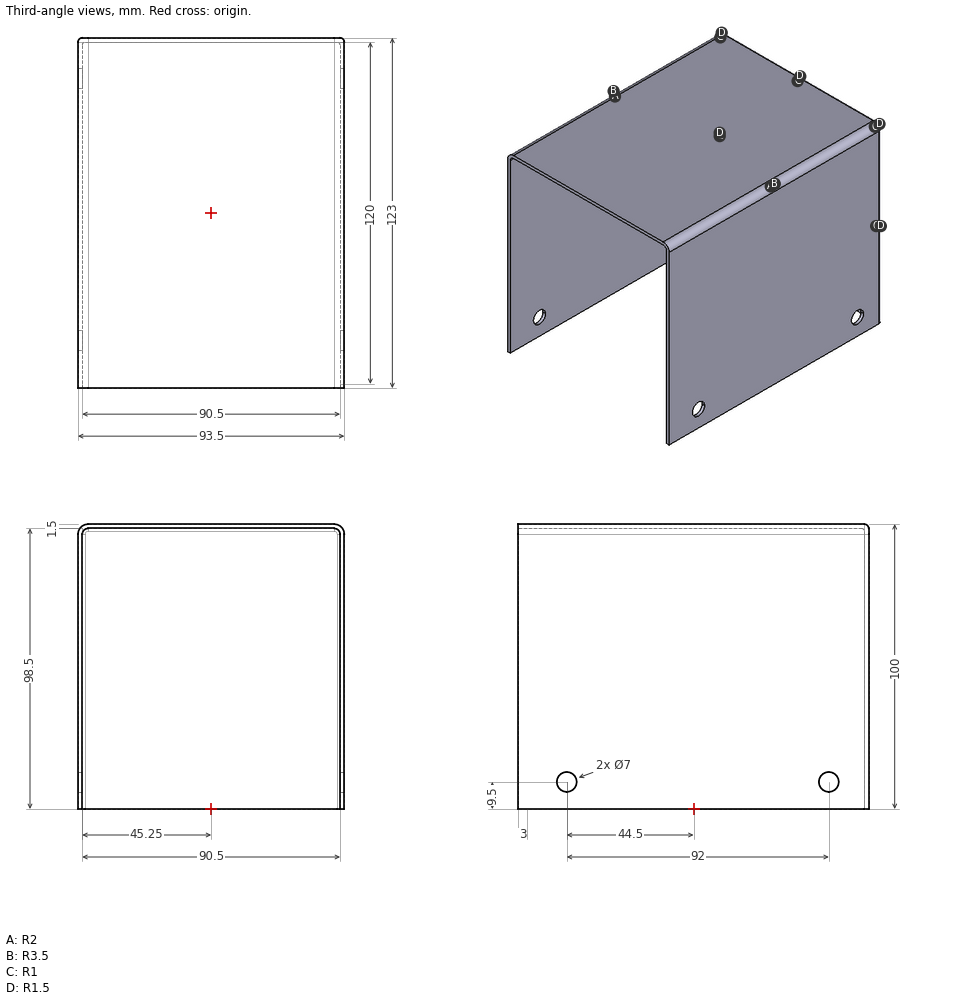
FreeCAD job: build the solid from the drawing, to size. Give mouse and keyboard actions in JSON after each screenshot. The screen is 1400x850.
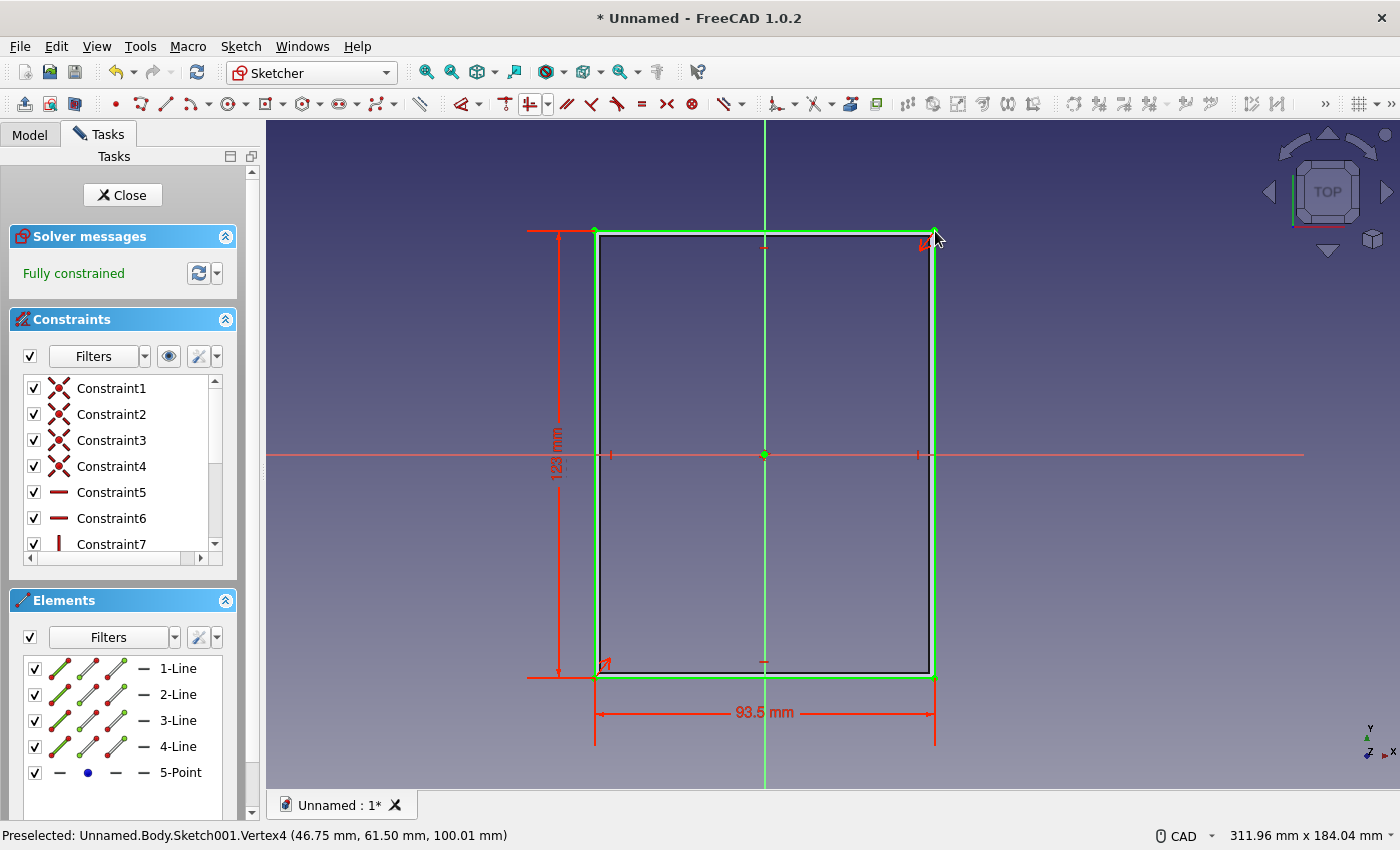
{"action": "left_click", "coordinate": [123, 195]}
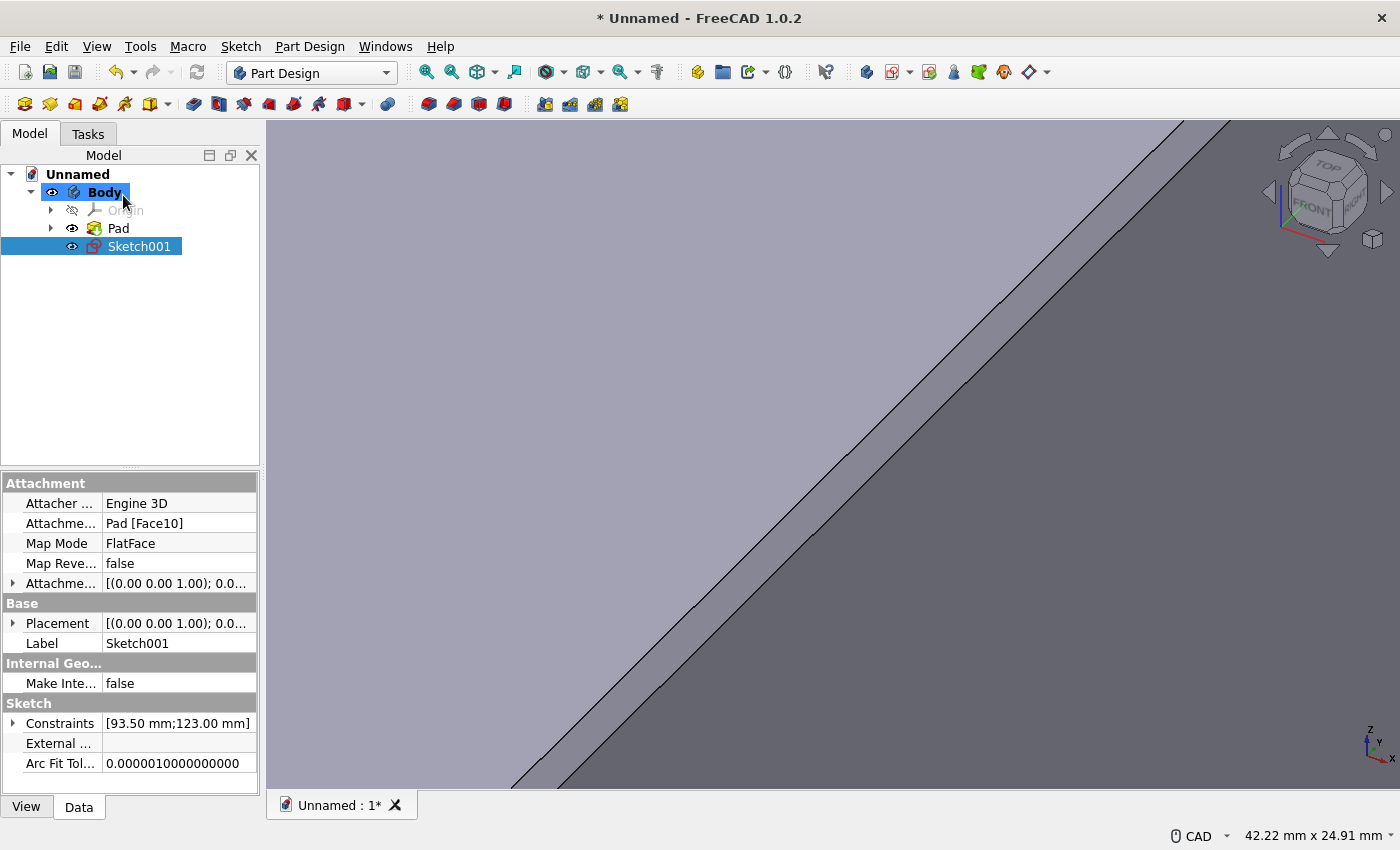
{"action": "left_click", "coordinate": [25, 104]}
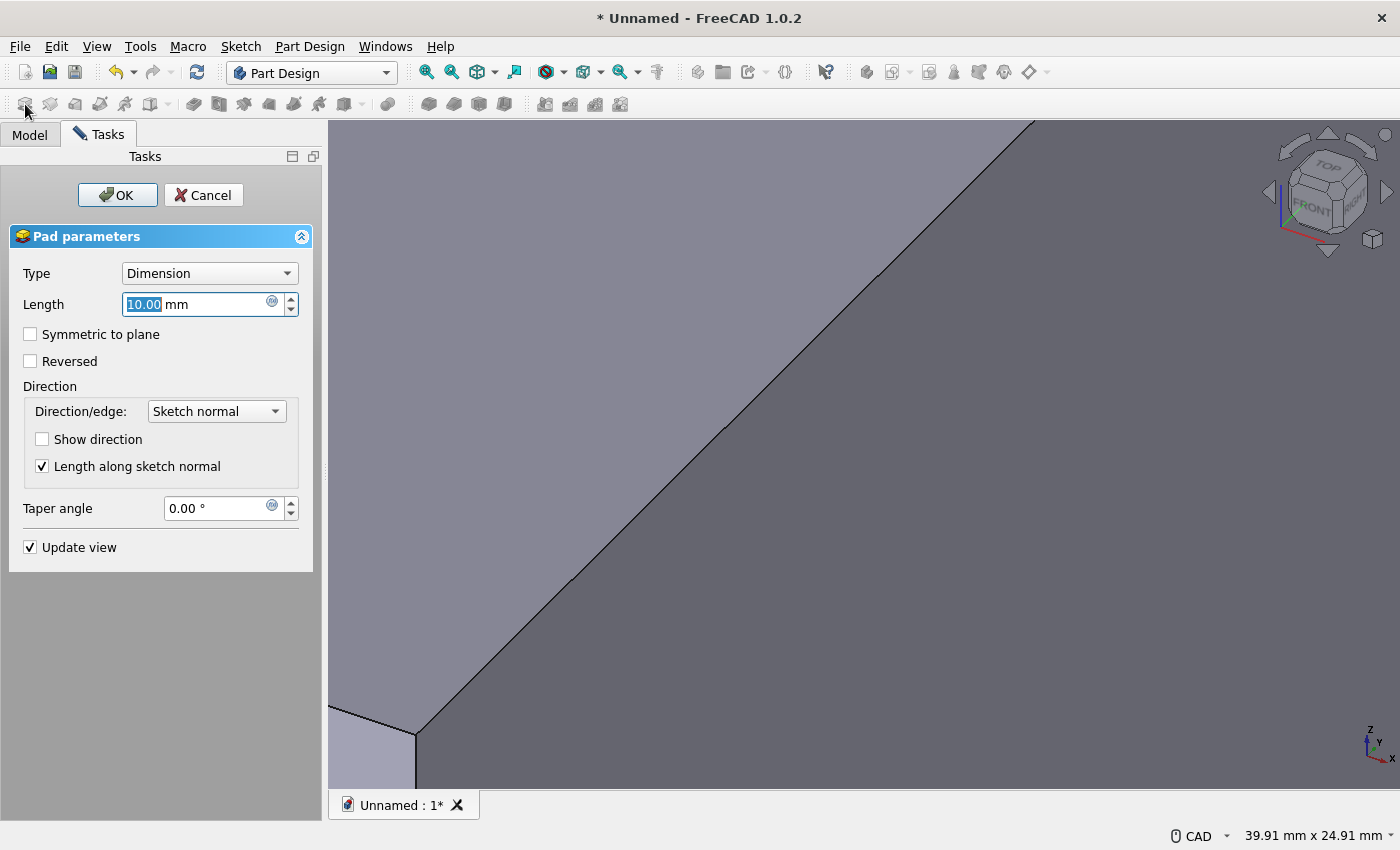
{"action": "type", "text": "1.5"}
{"action": "key", "text": "Tab"}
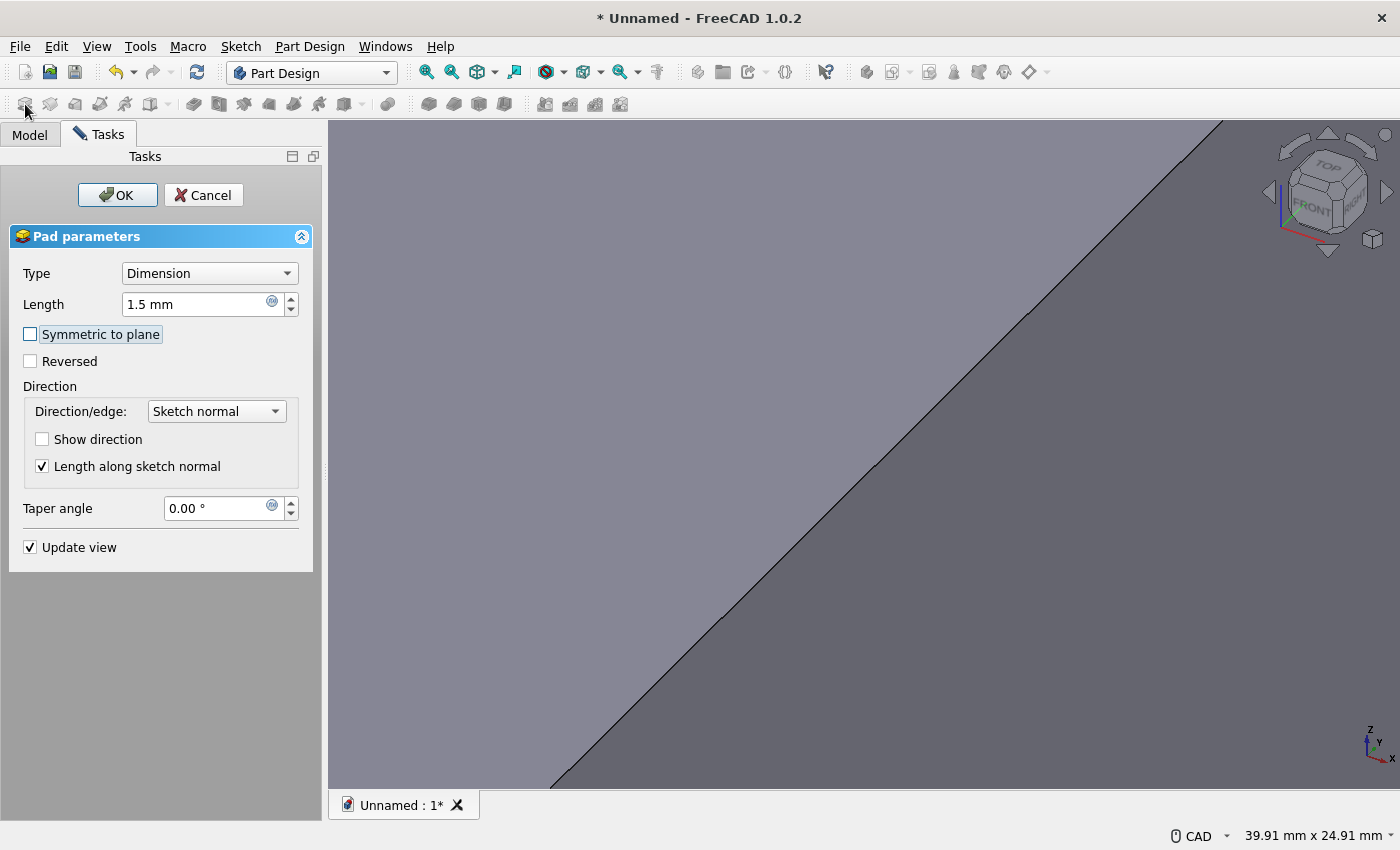
{"action": "left_click", "coordinate": [31, 361]}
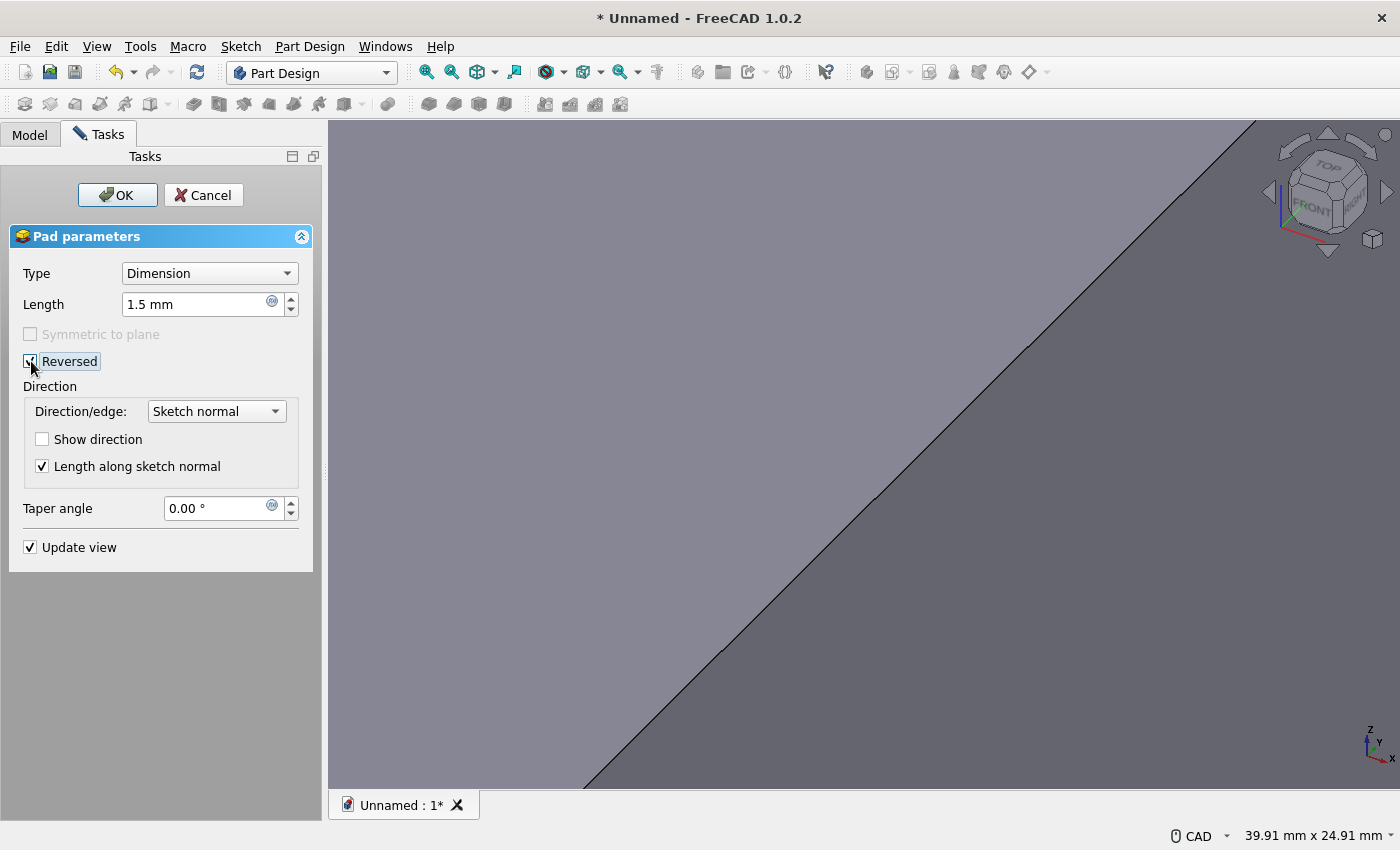
{"action": "left_click", "coordinate": [118, 195]}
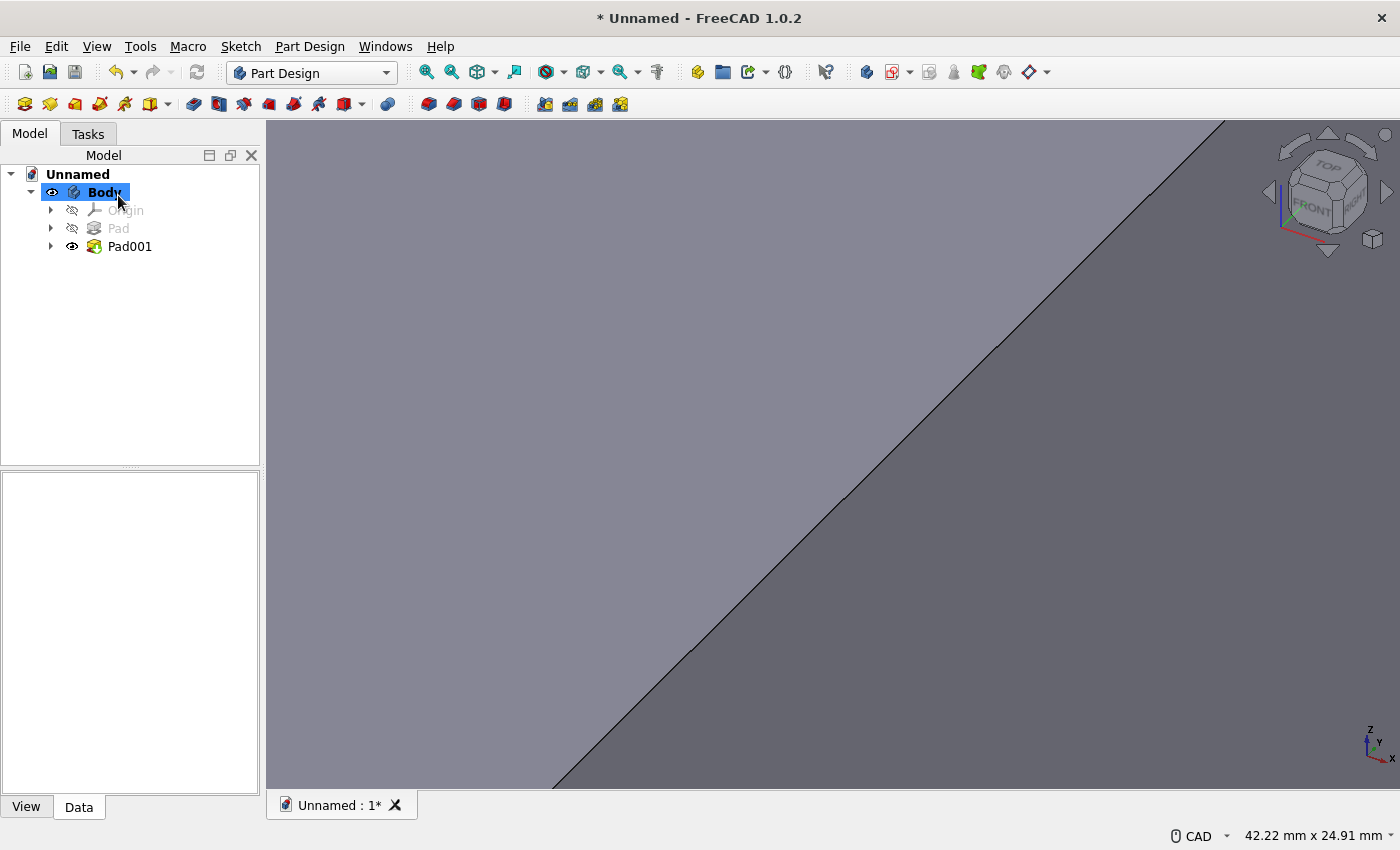
{"action": "left_click", "coordinate": [427, 72]}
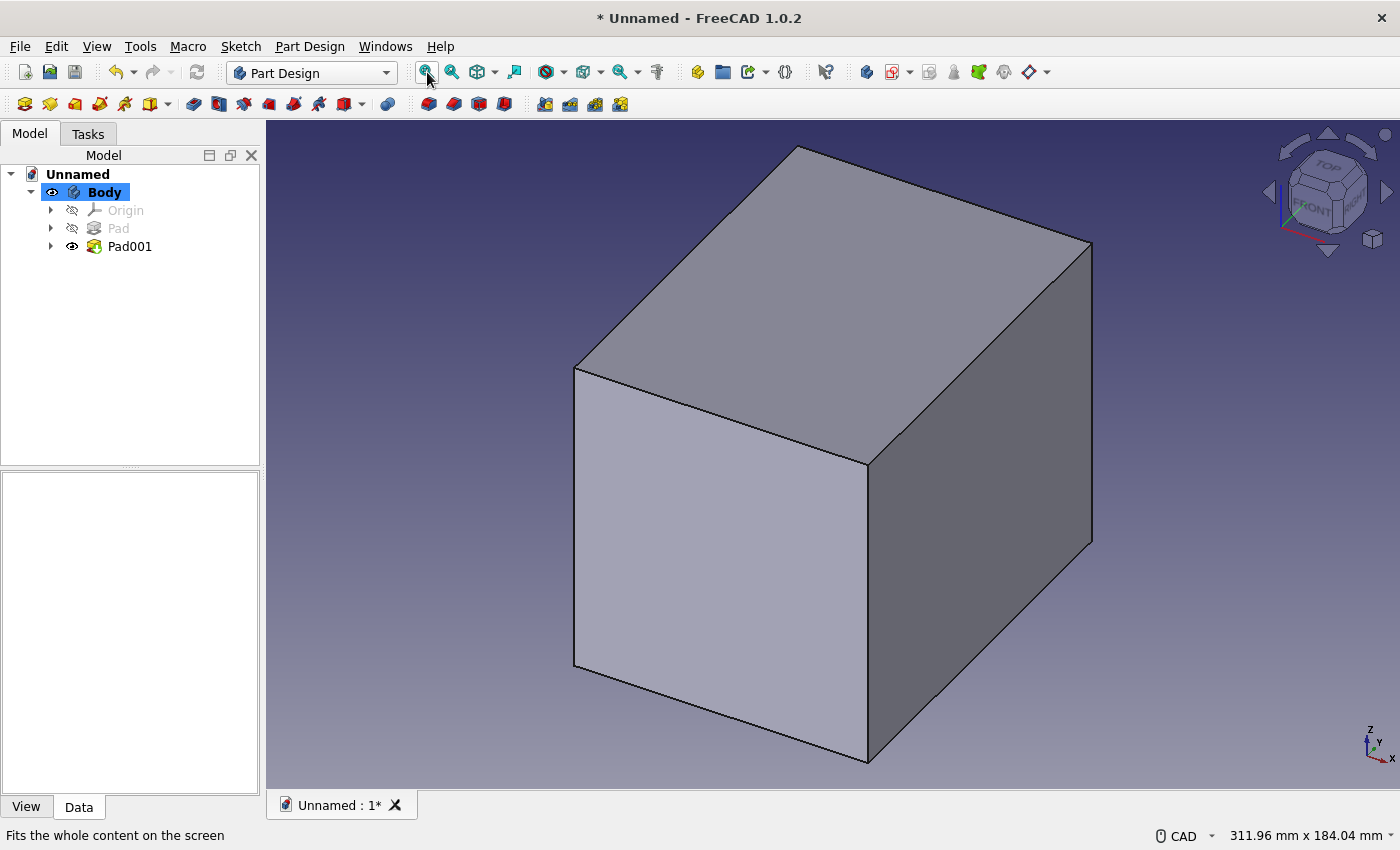
{"action": "left_click", "coordinate": [721, 565]}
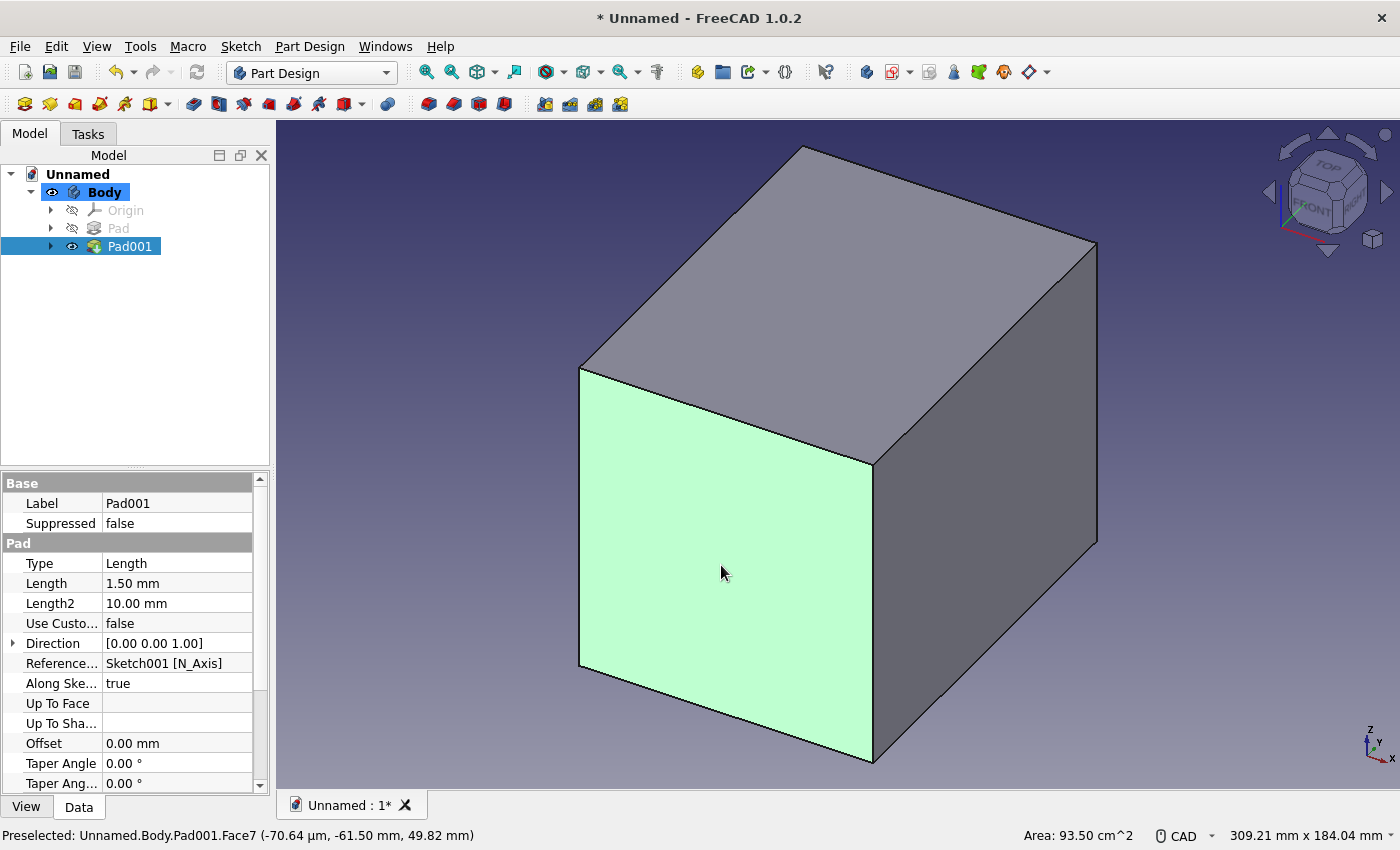
{"action": "left_click", "coordinate": [892, 72]}